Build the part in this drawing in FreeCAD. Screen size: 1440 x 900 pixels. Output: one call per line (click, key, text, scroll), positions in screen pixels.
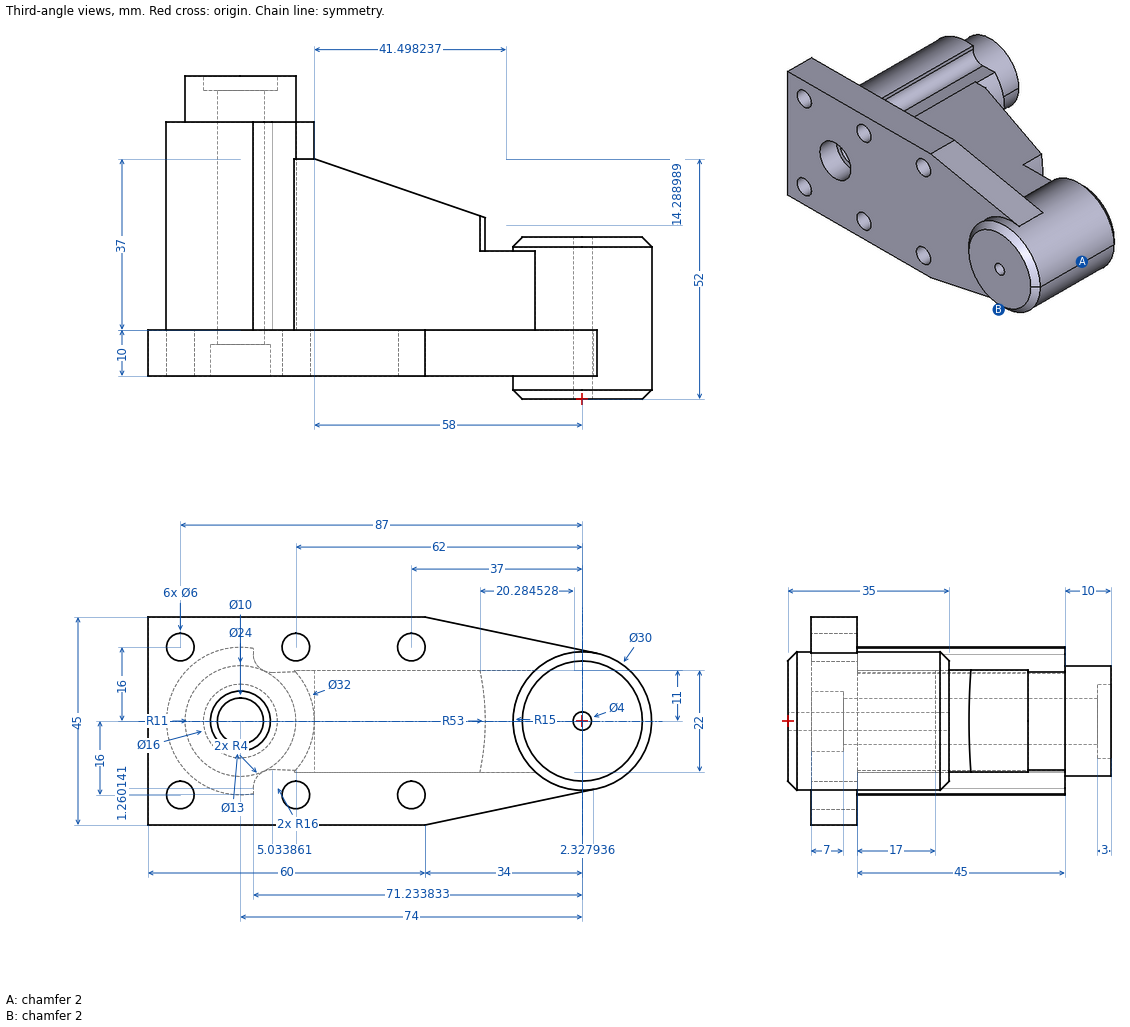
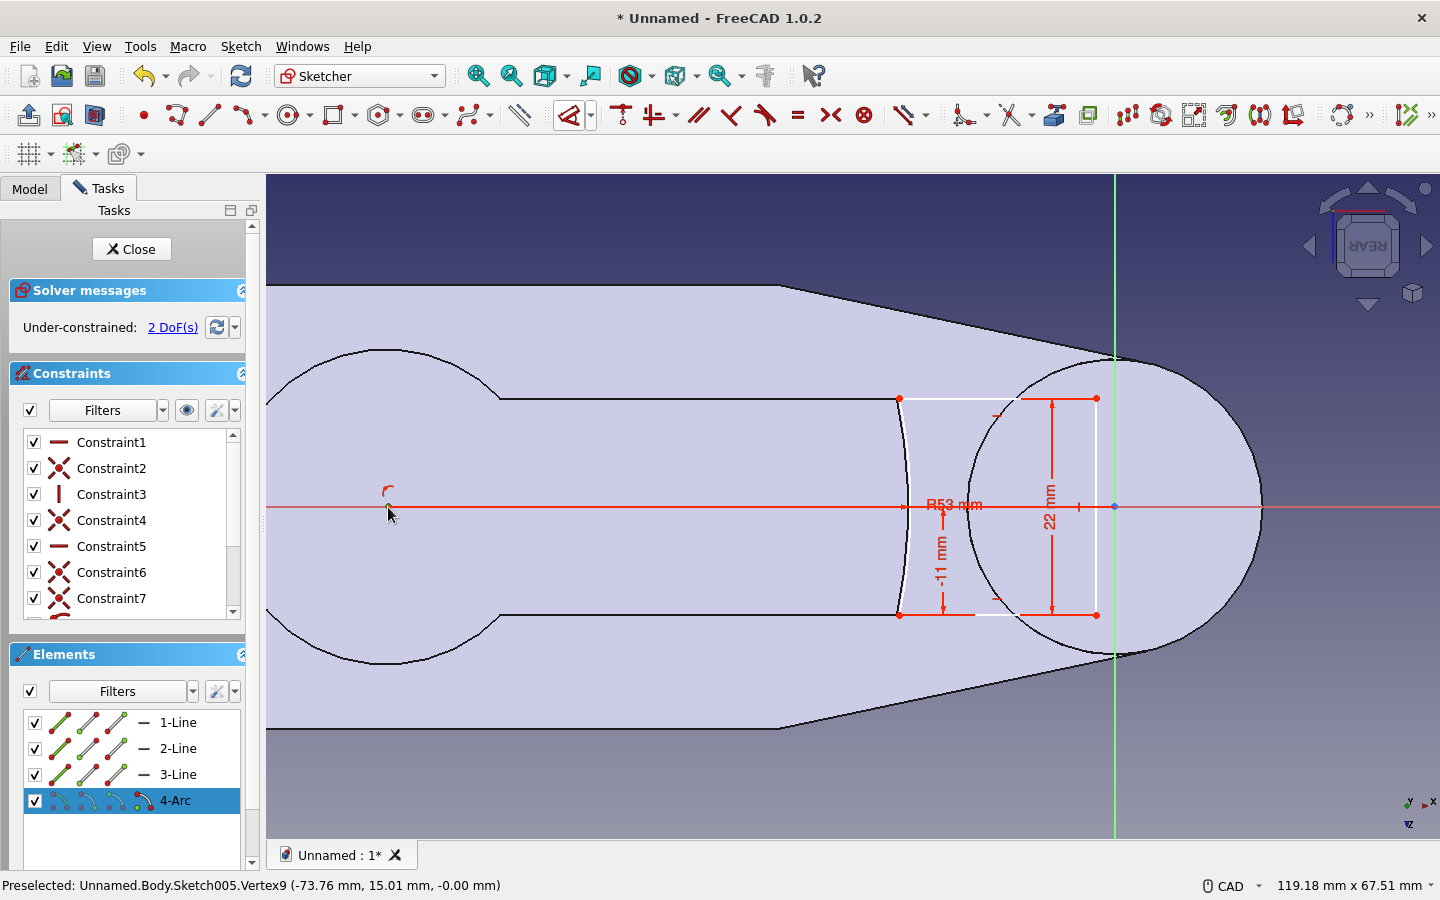
click(590, 116)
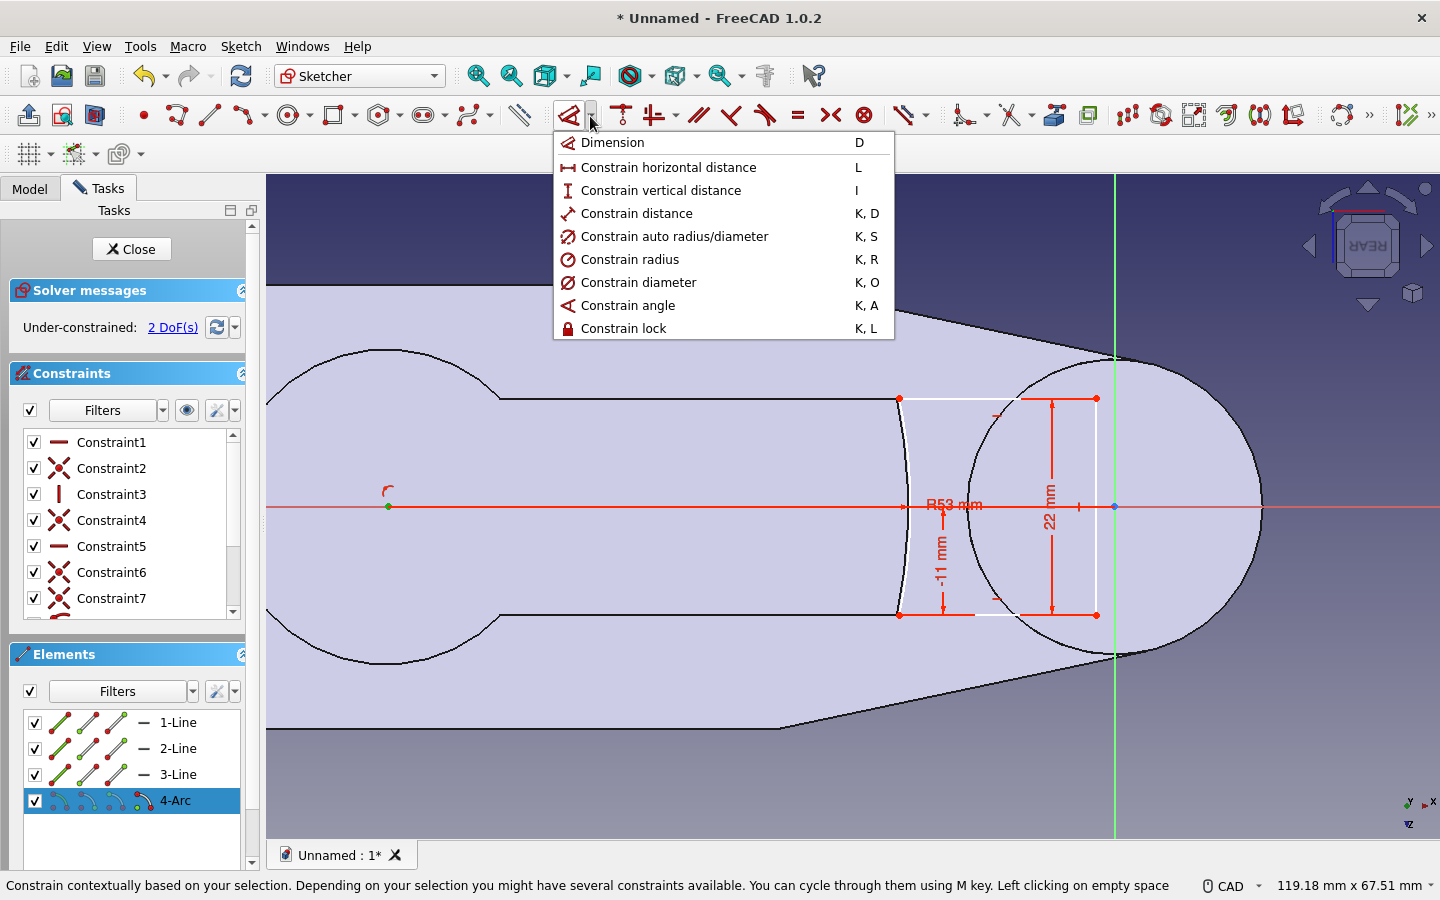
click(724, 168)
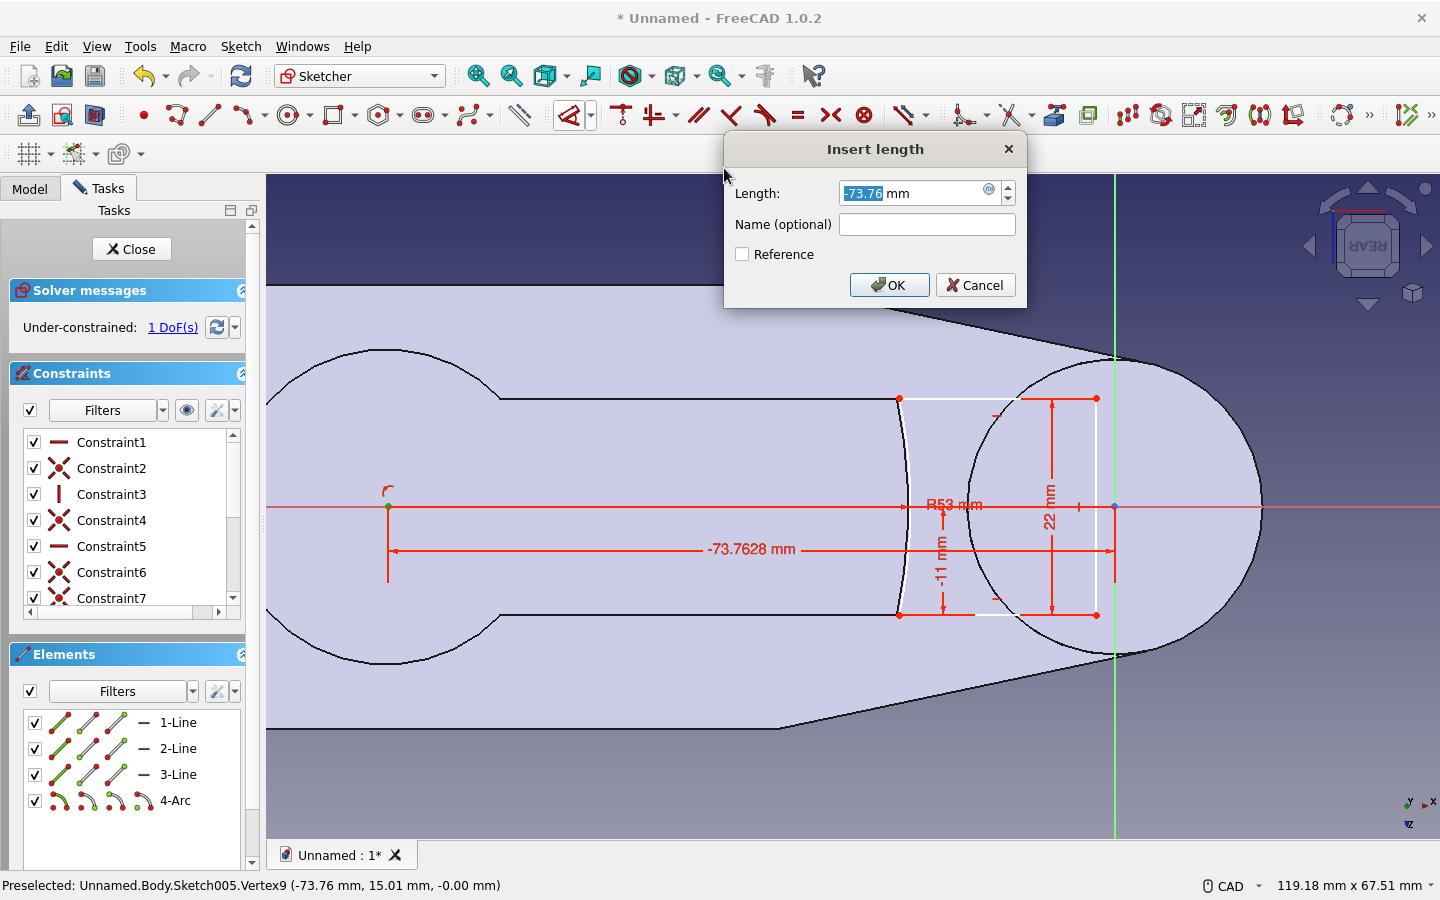
text(-74)
key(Return)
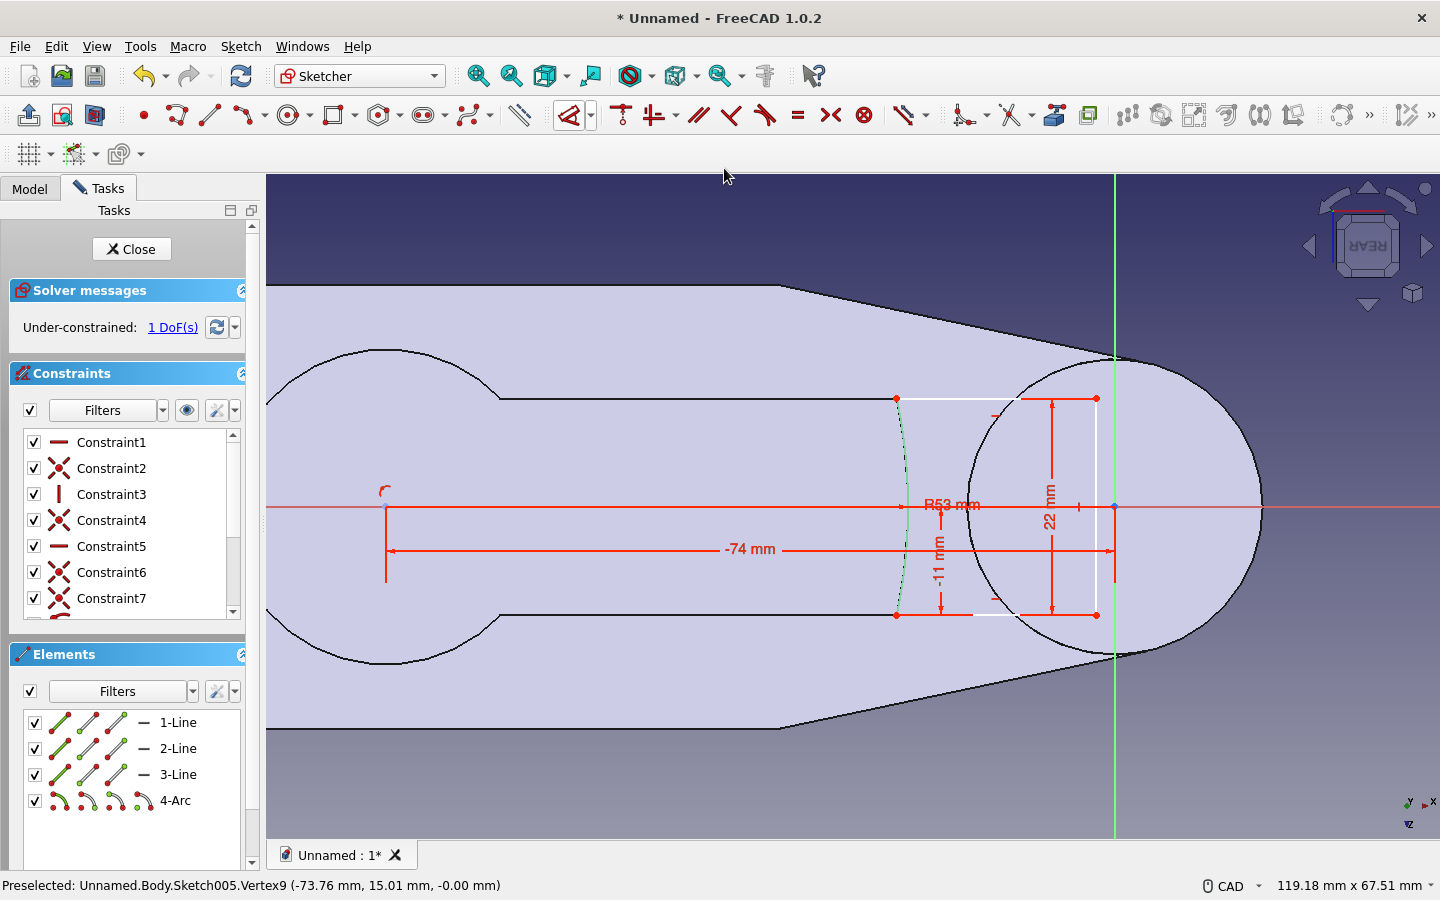
click(957, 615)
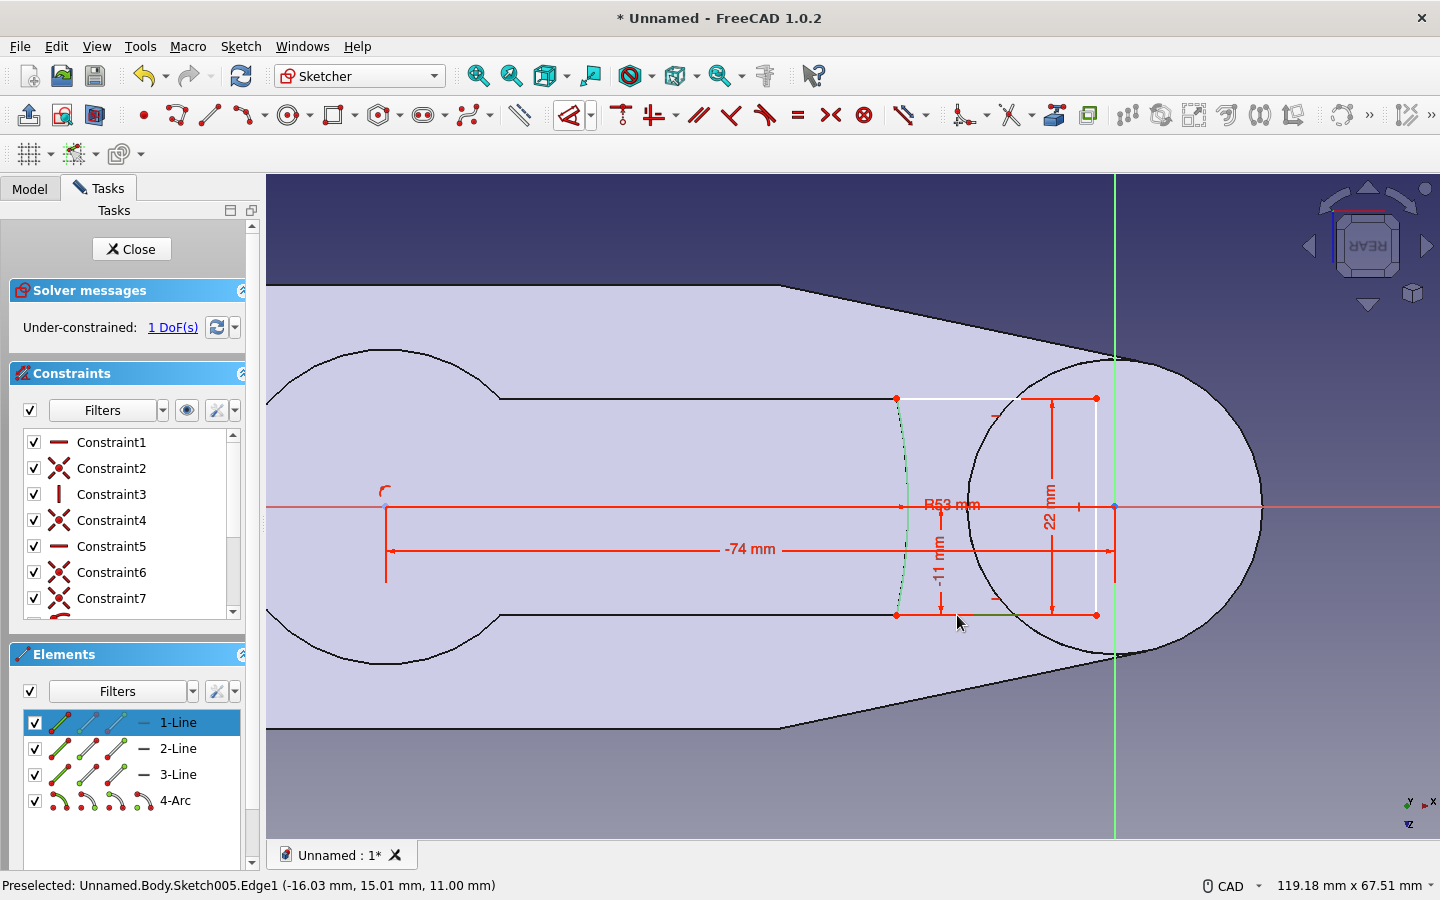
key(l)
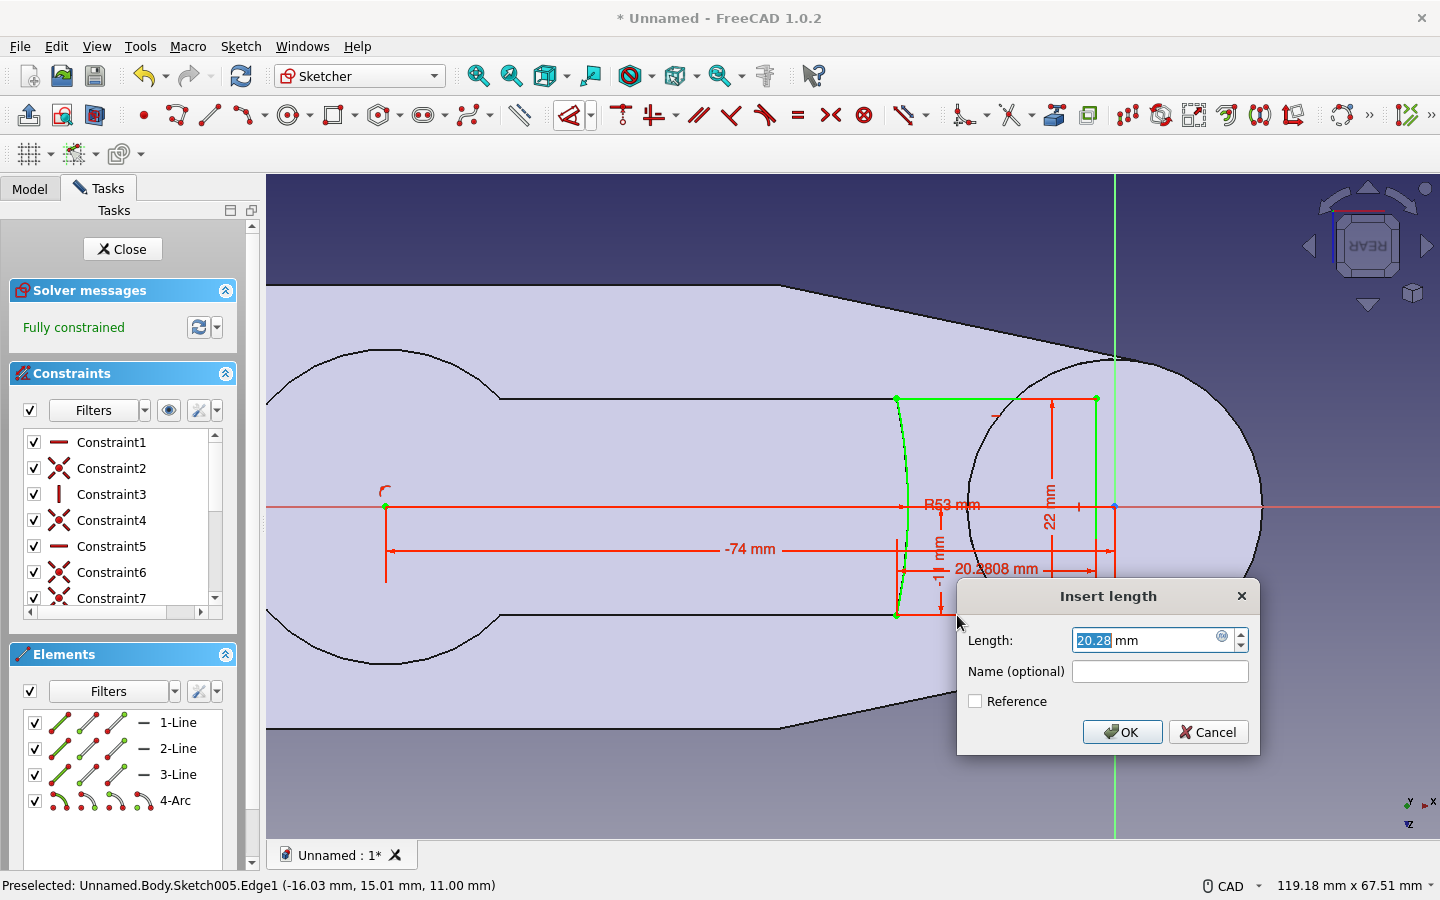
text(20.284528)
key(Return)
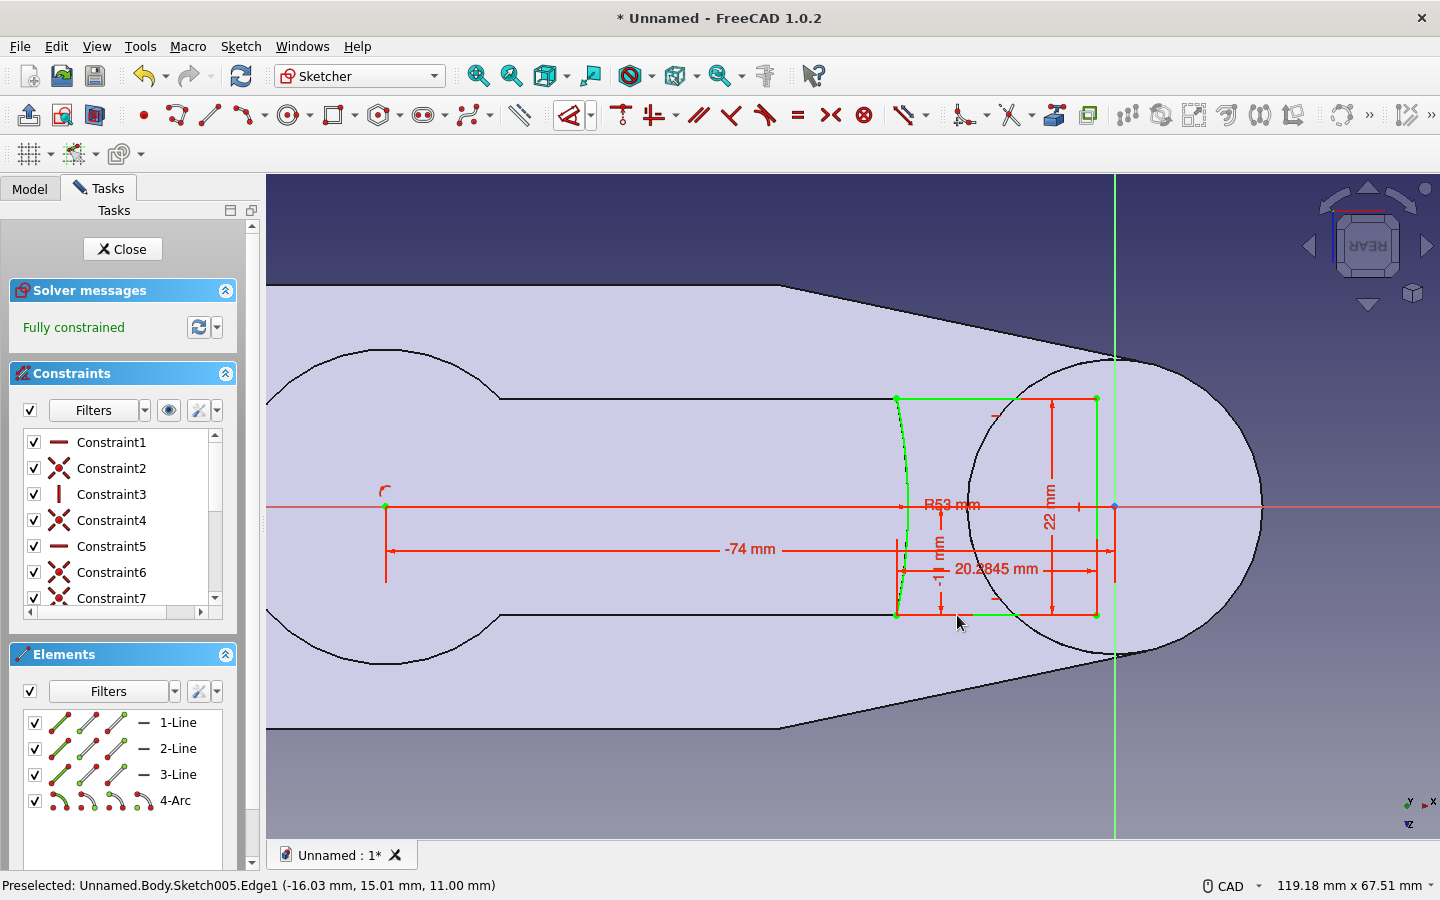
click(123, 249)